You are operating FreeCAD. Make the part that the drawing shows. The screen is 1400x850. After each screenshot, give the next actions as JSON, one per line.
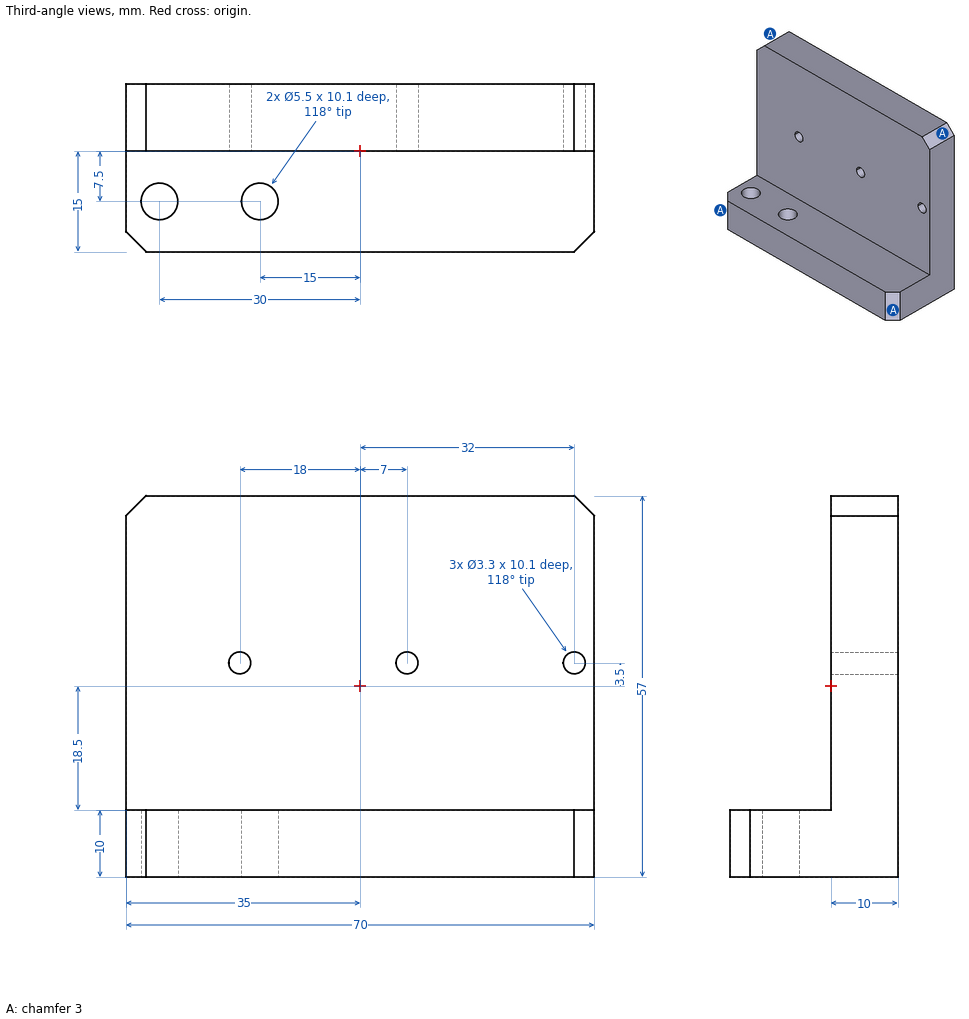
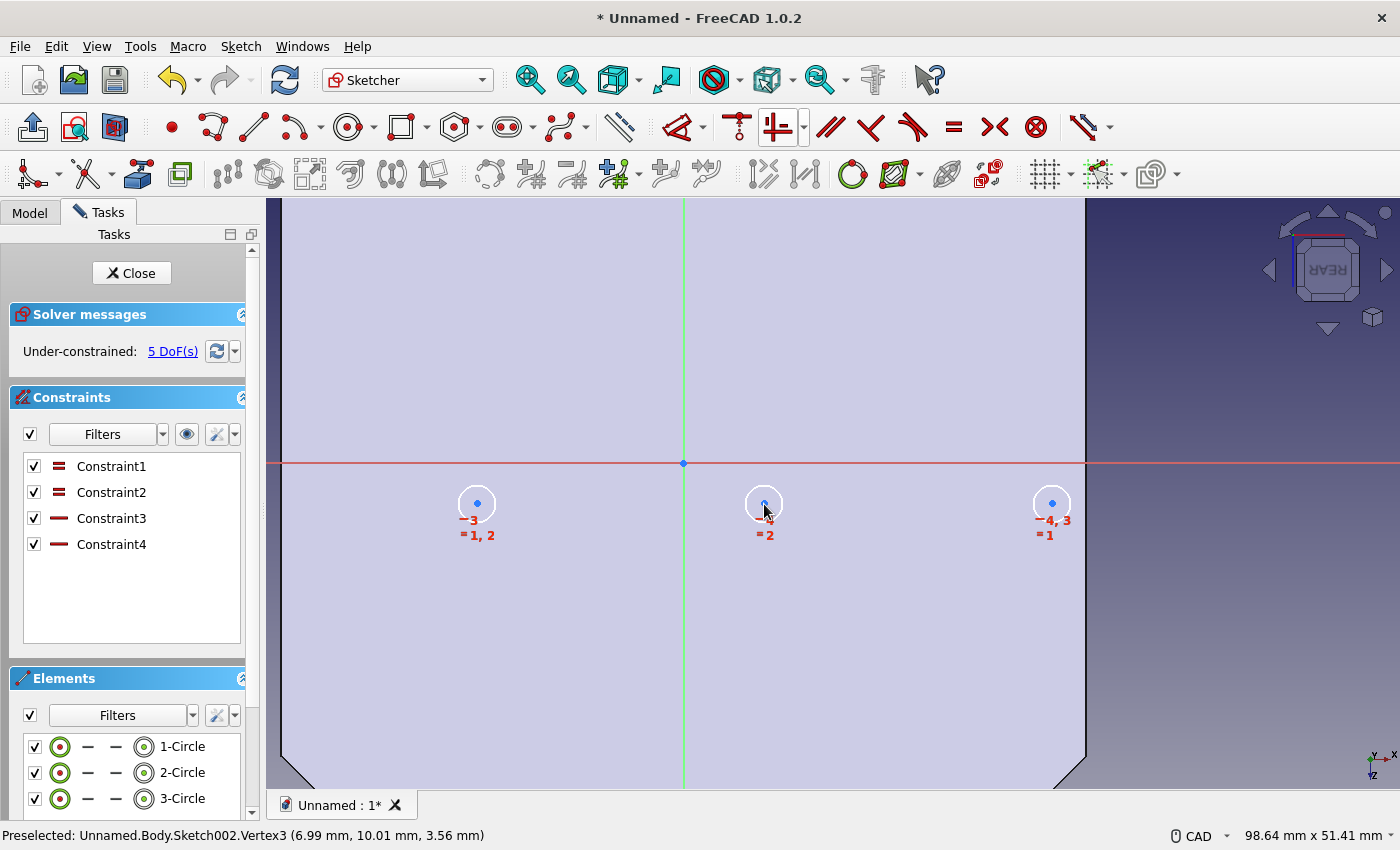
{"action": "left_click", "coordinate": [676, 128]}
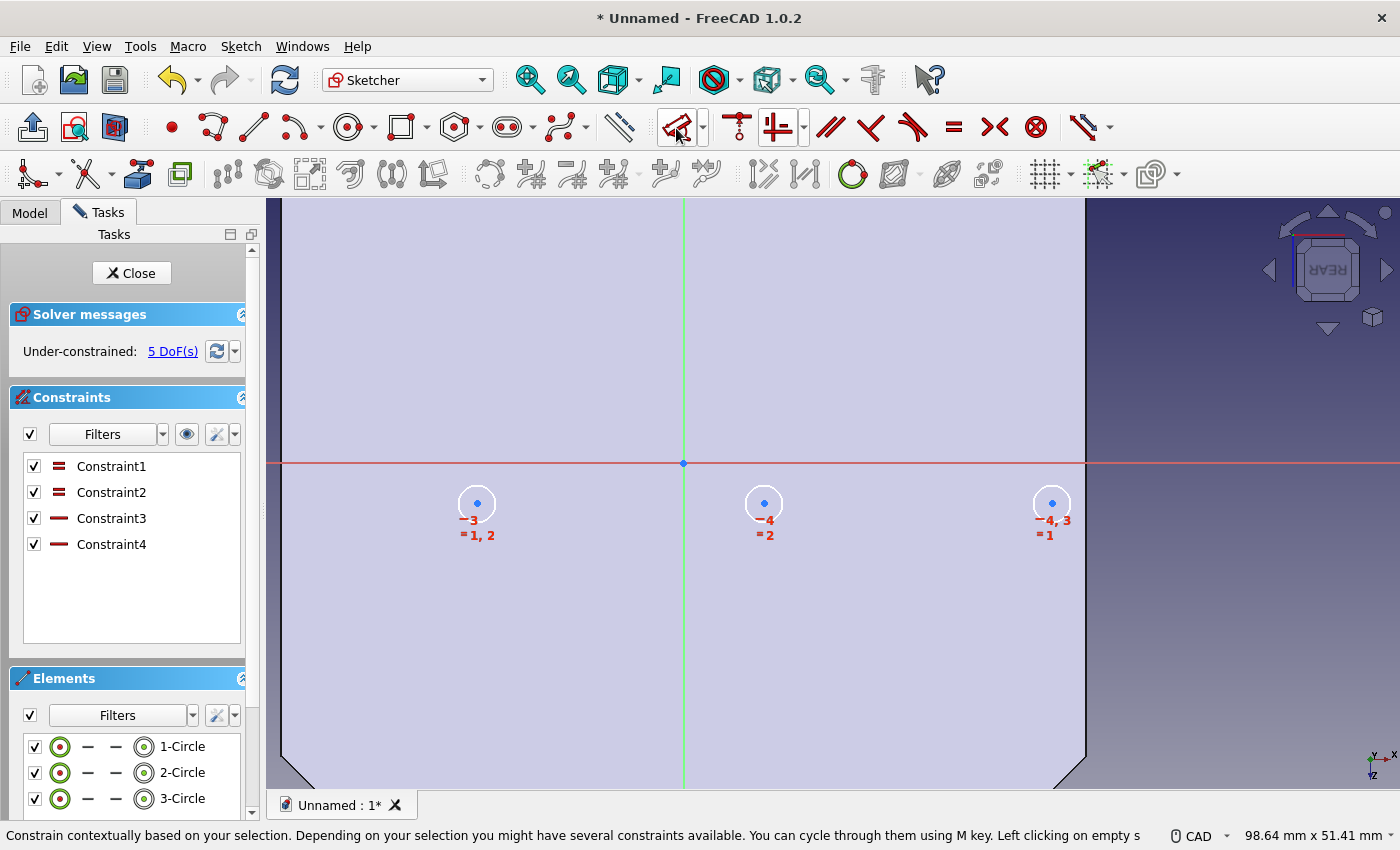
{"action": "left_click", "coordinate": [1065, 491]}
{"action": "left_click", "coordinate": [1100, 490]}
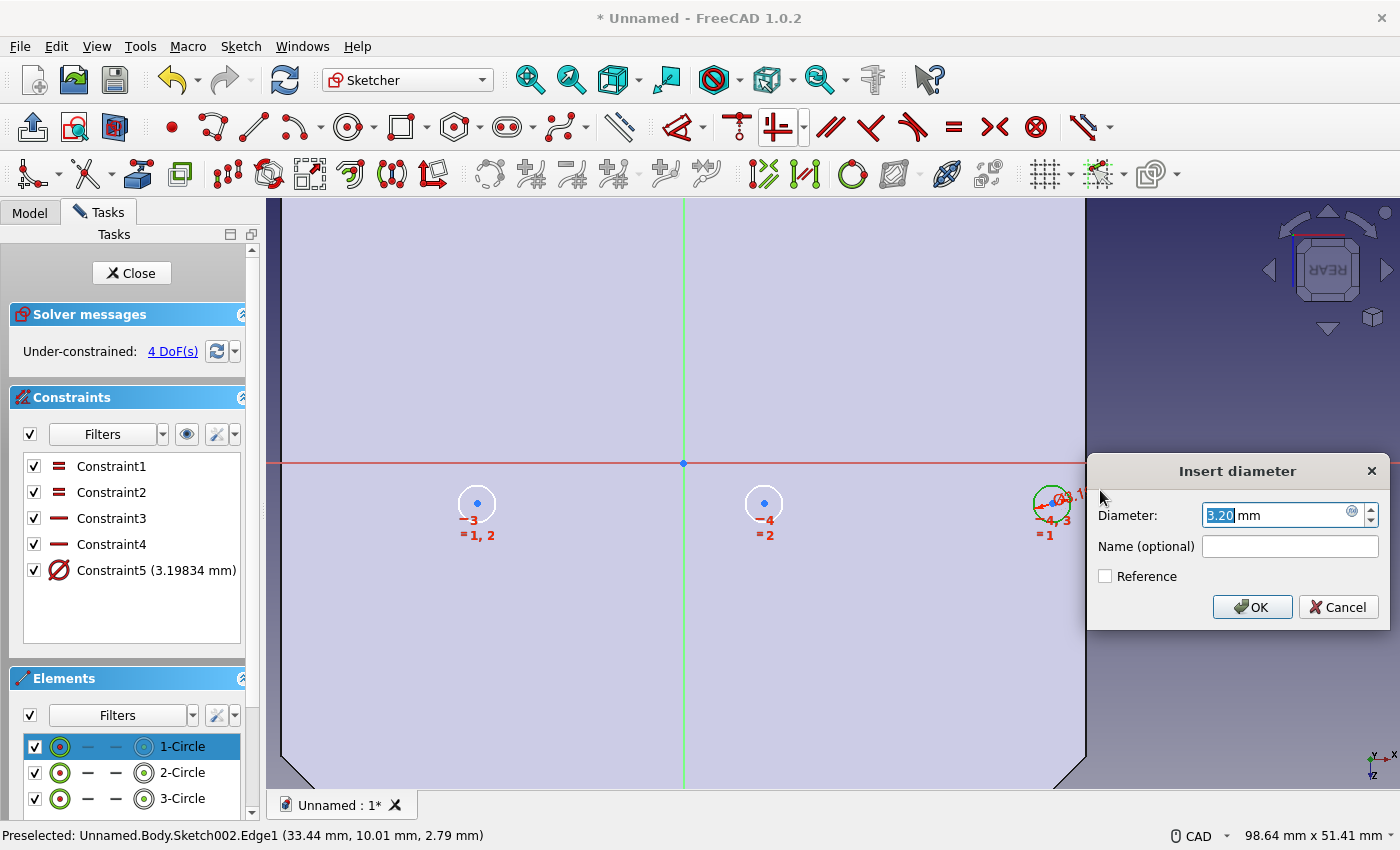
{"action": "type", "text": "3.3"}
{"action": "key", "text": "Return"}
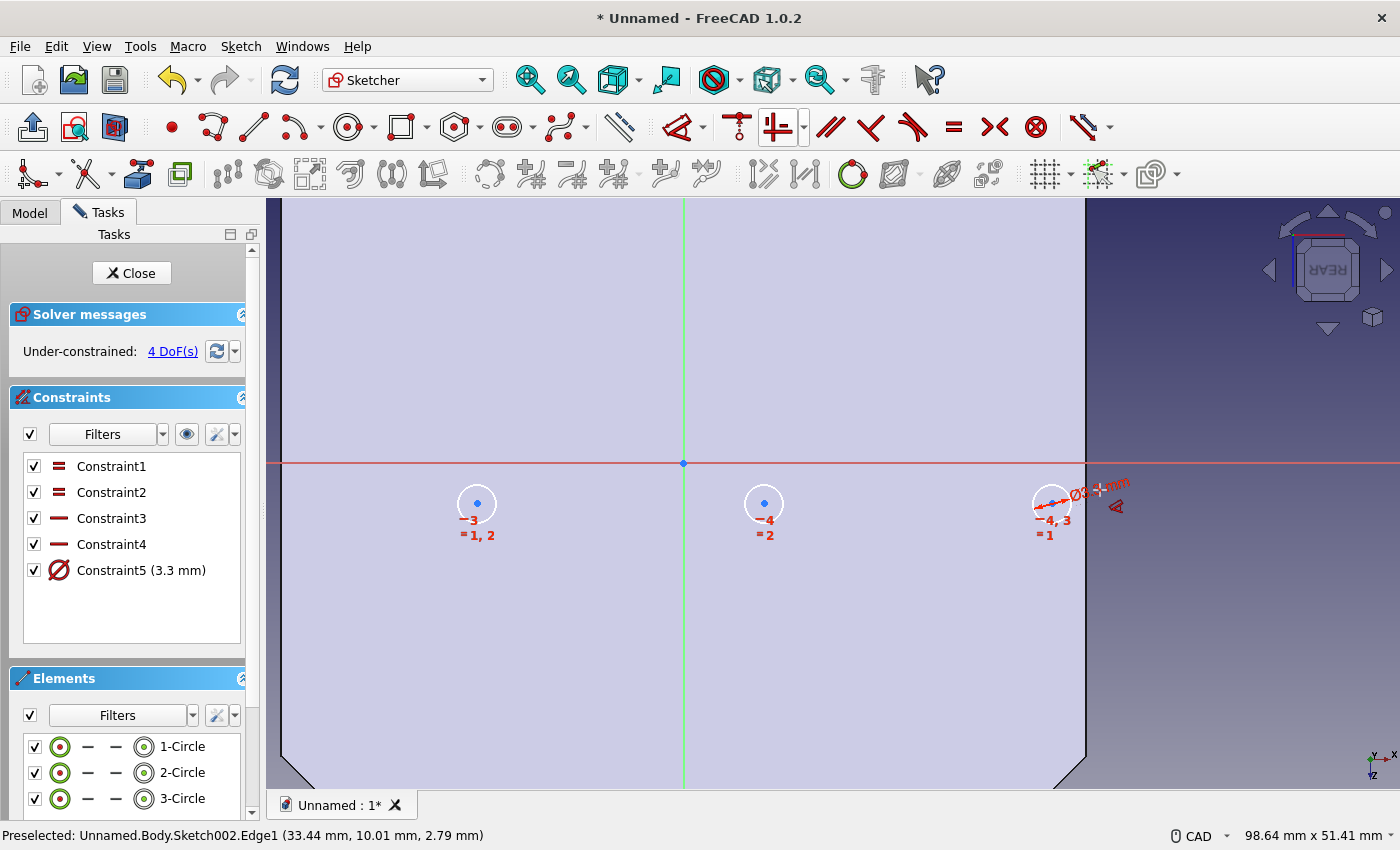
{"action": "left_click", "coordinate": [764, 504]}
{"action": "left_click", "coordinate": [724, 429]}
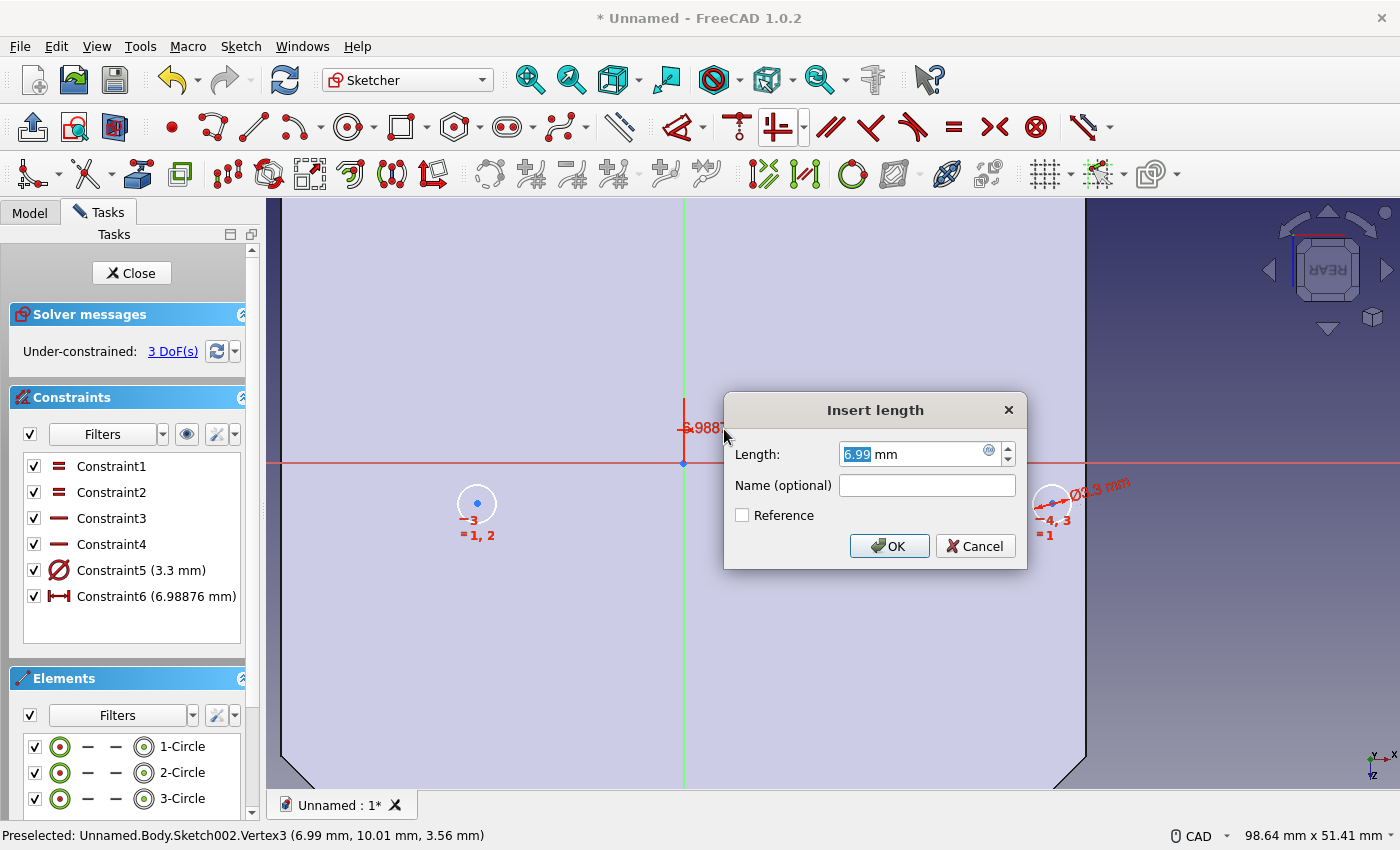
{"action": "type", "text": "7"}
{"action": "key", "text": "Return"}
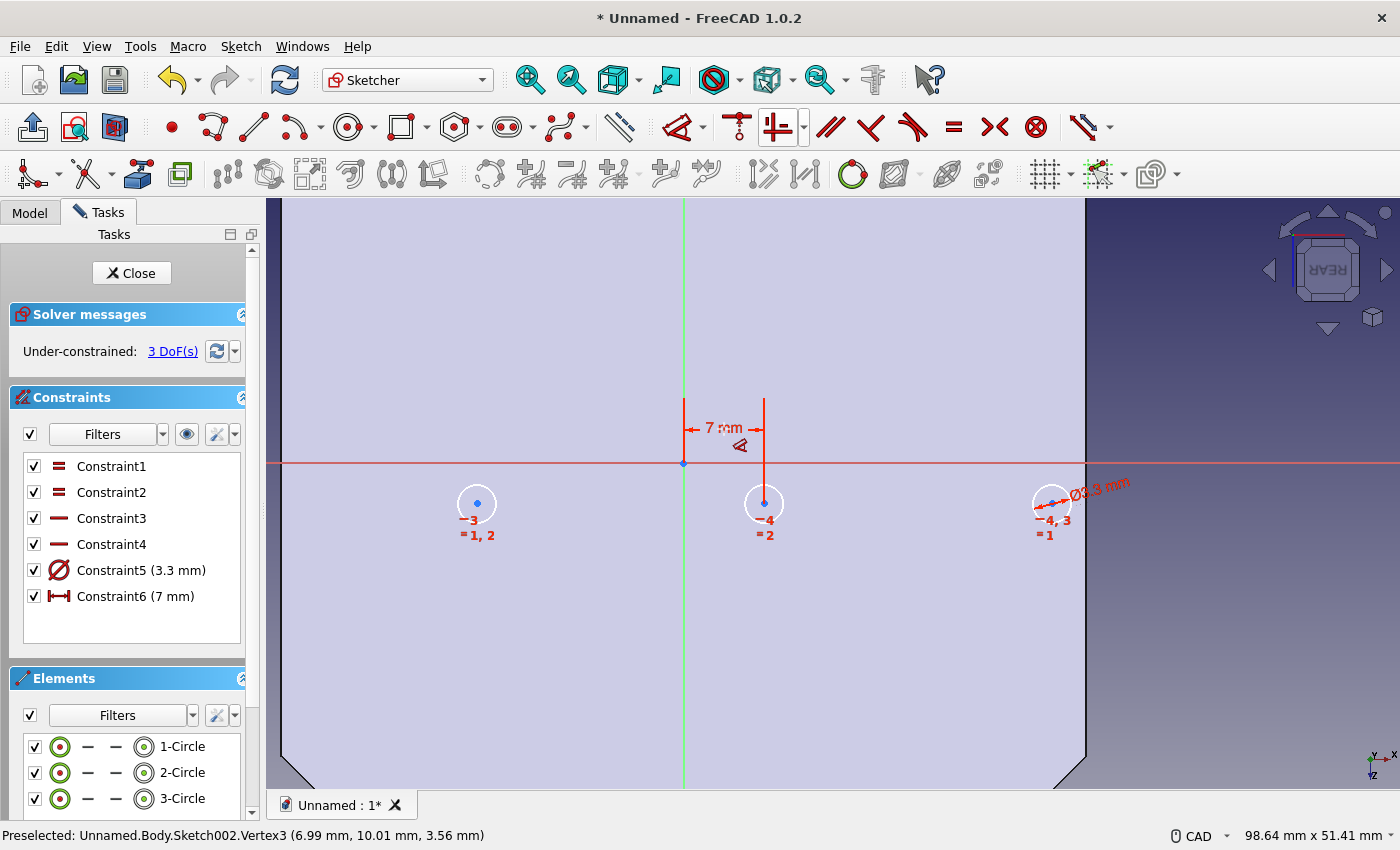
{"action": "left_click", "coordinate": [1052, 504]}
{"action": "left_click", "coordinate": [868, 429]}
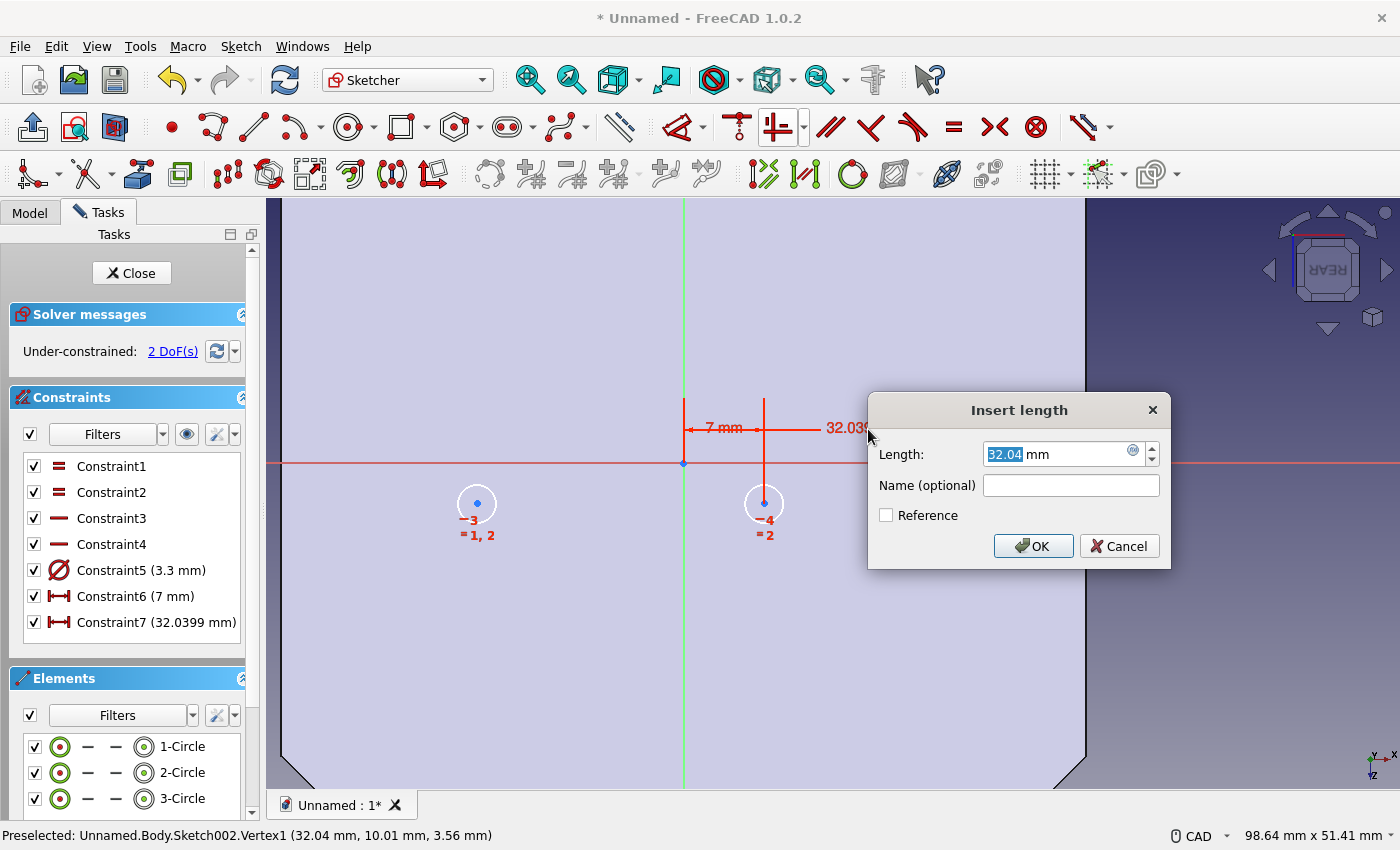
{"action": "type", "text": "32"}
{"action": "key", "text": "Return"}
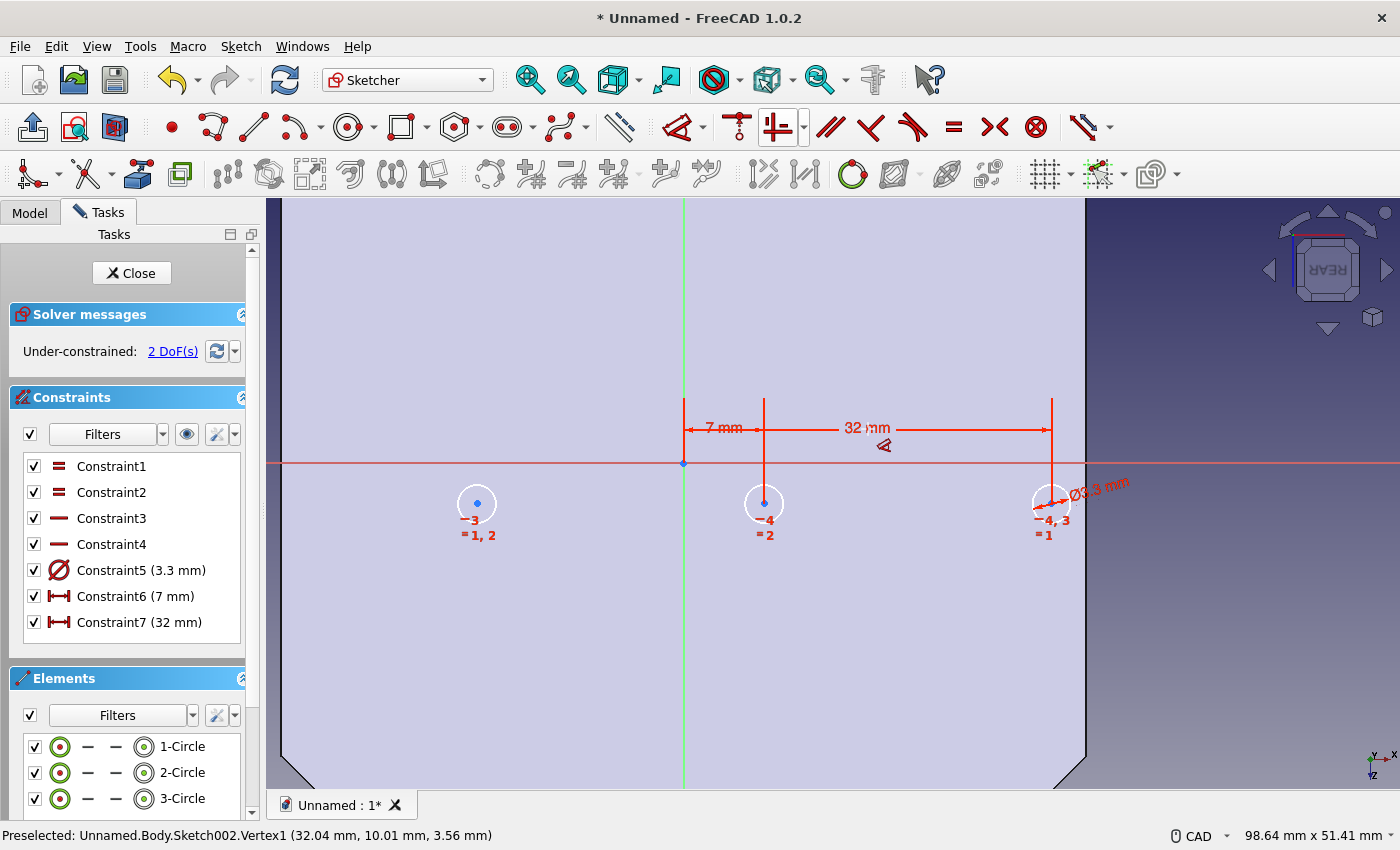
{"action": "left_click", "coordinate": [477, 504]}
{"action": "left_click", "coordinate": [580, 429]}